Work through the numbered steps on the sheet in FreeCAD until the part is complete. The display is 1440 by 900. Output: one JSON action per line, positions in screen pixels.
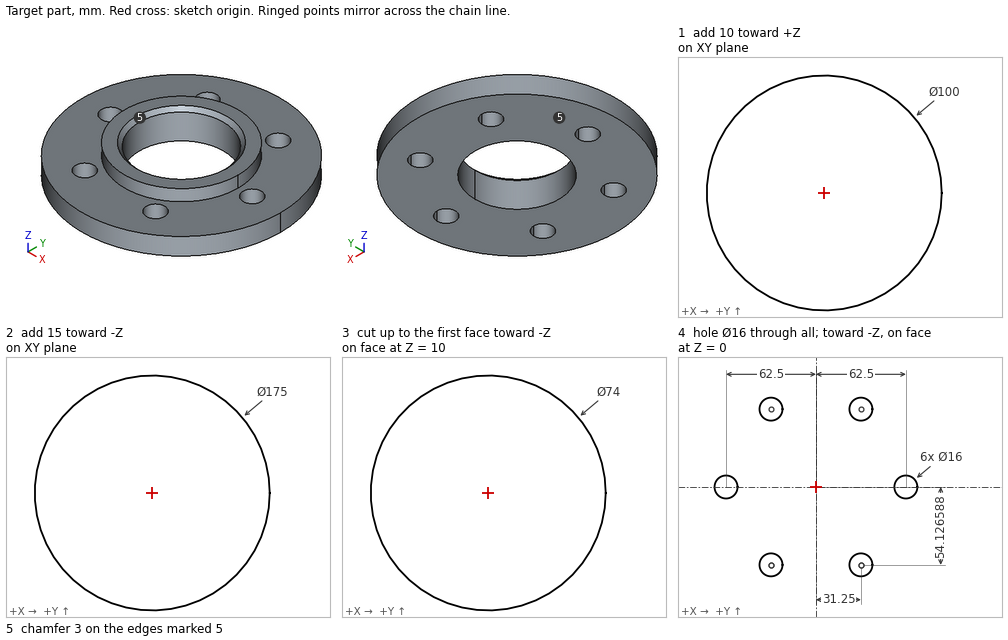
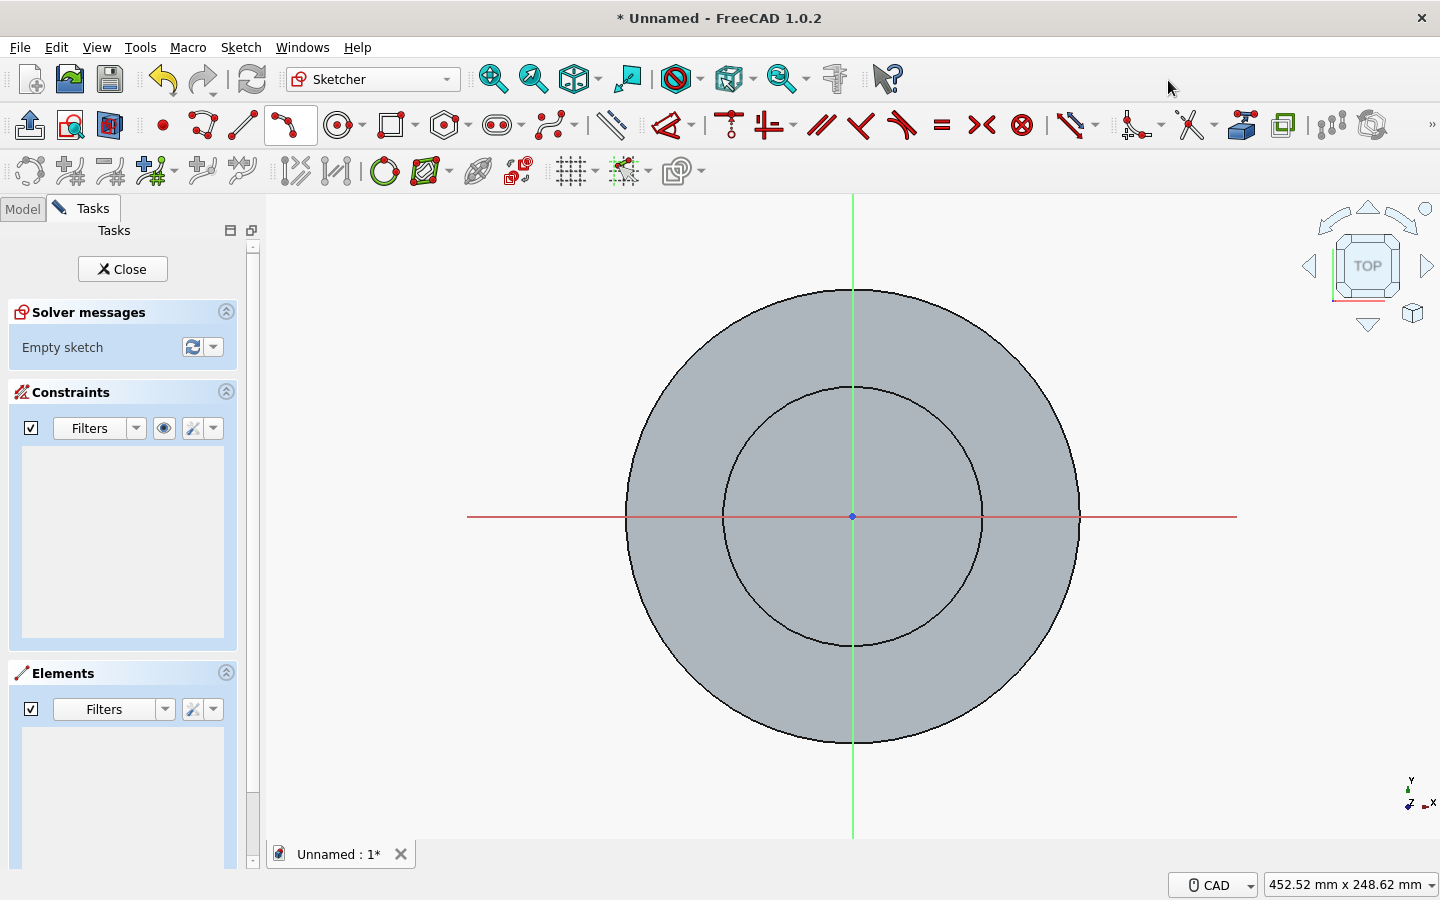
{"action": "scroll", "coordinate": [909, 517], "scroll_direction": "up", "scroll_amount": 4}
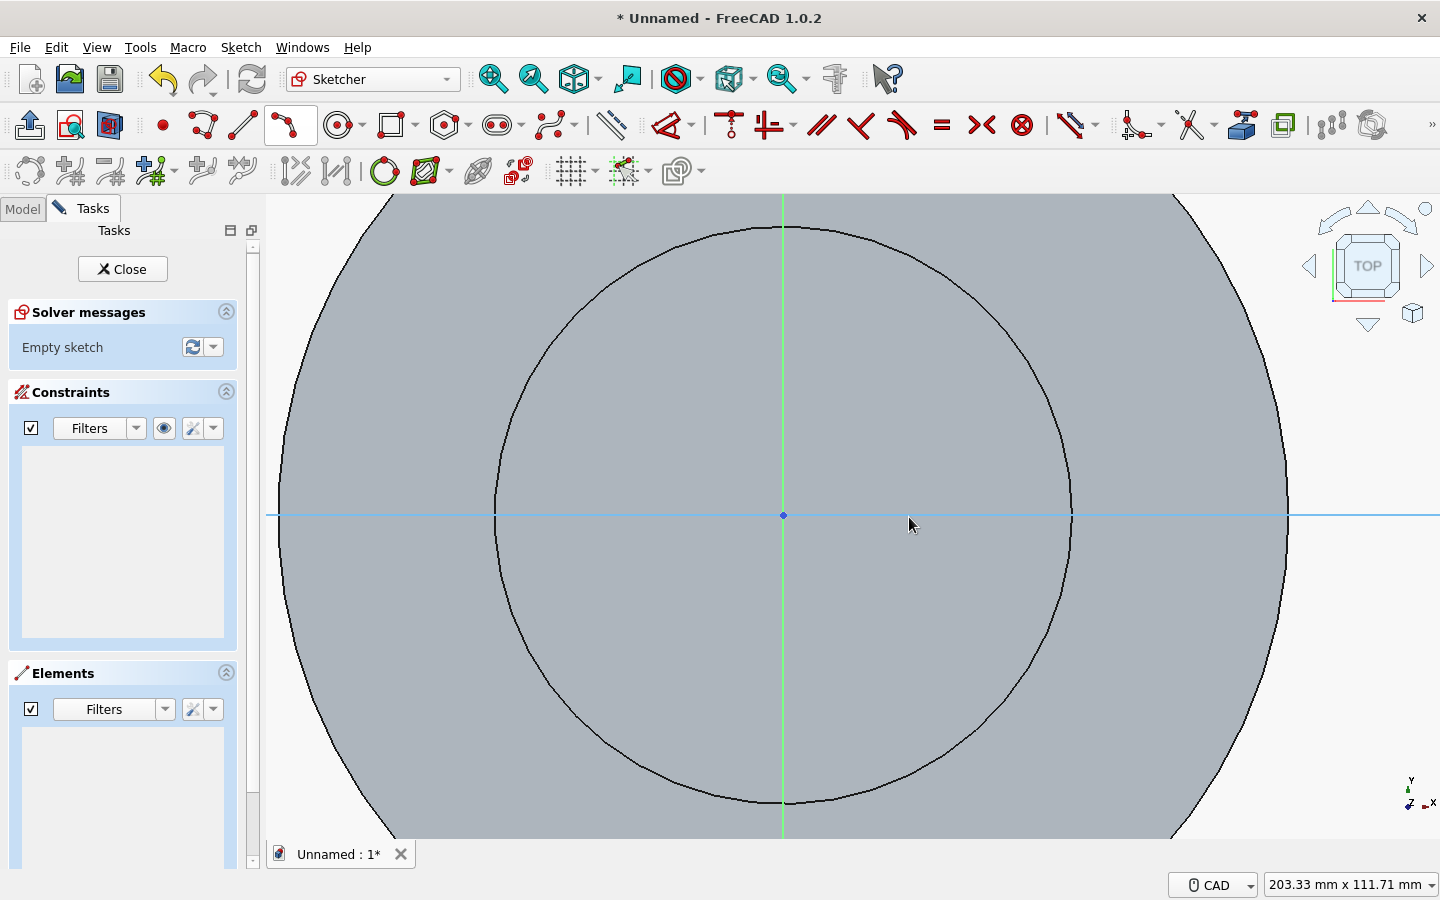
{"action": "left_click", "coordinate": [338, 126]}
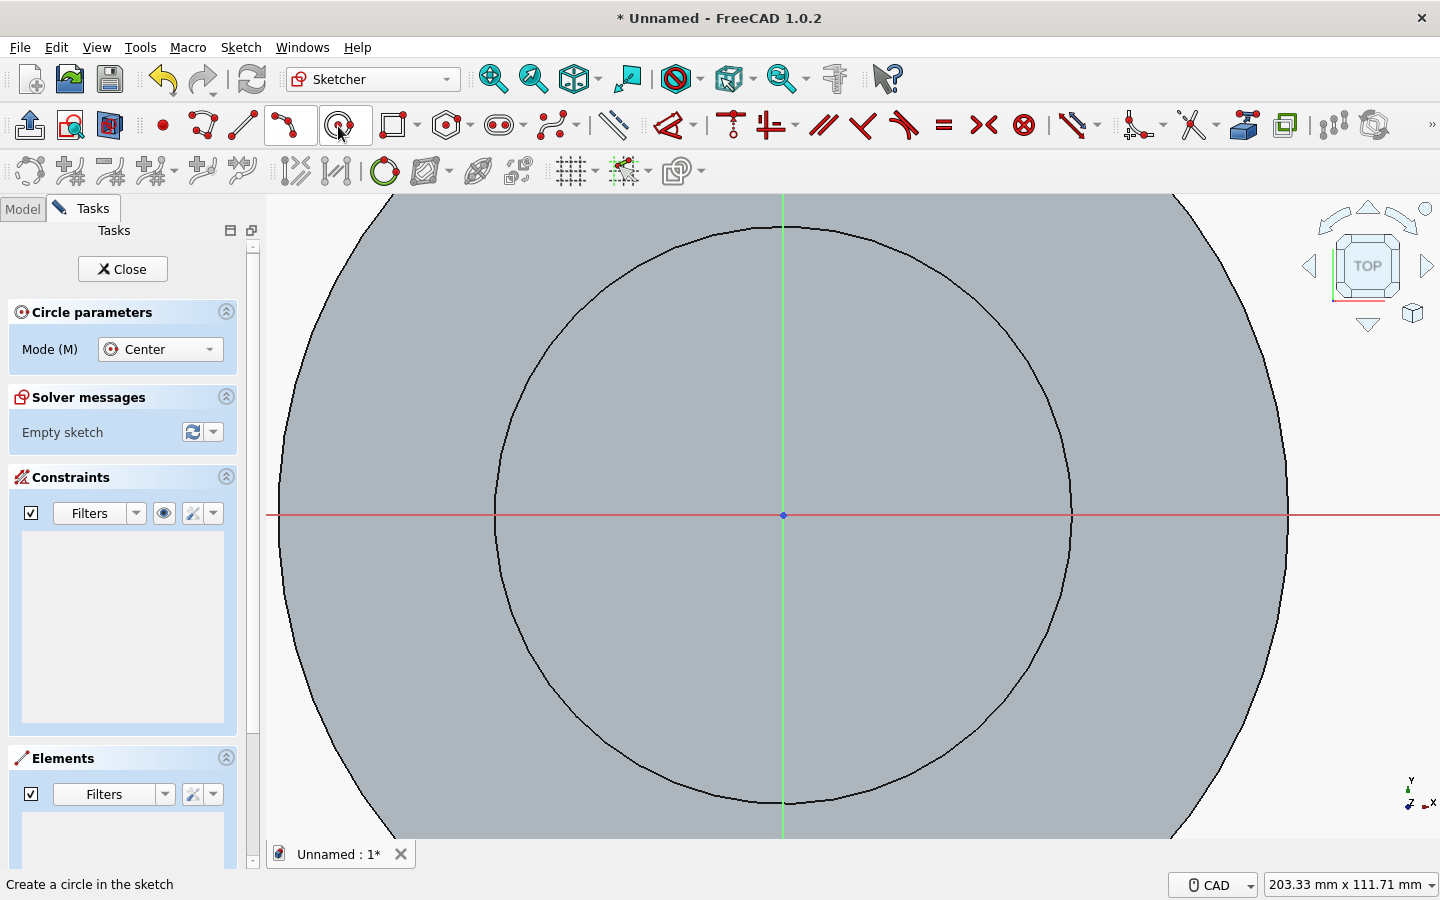
{"action": "left_click", "coordinate": [783, 515]}
{"action": "left_click", "coordinate": [934, 364]}
{"action": "key", "text": "Escape"}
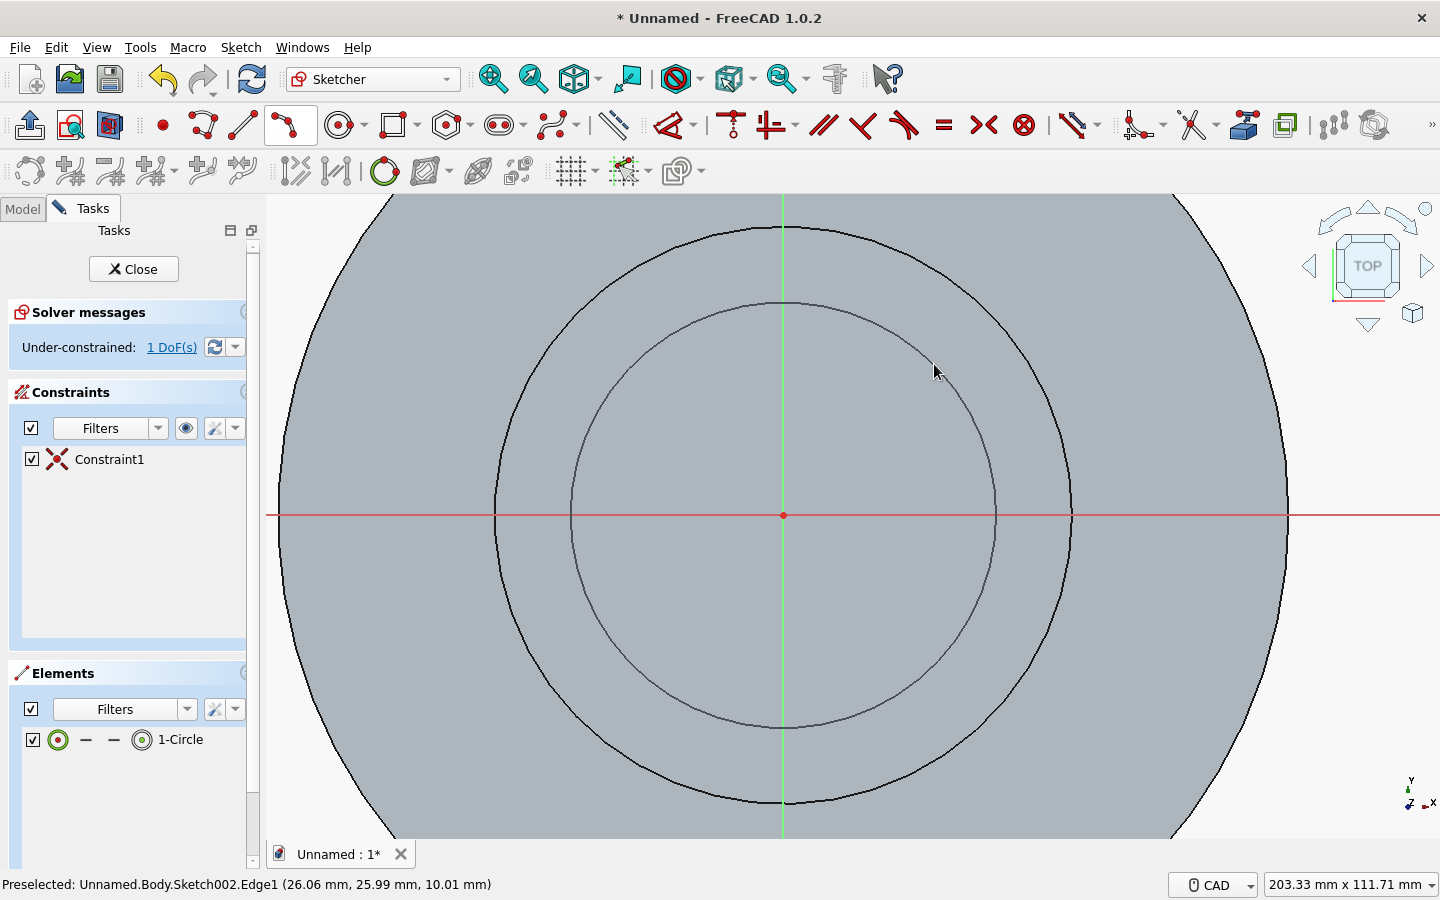
{"action": "left_click", "coordinate": [668, 126]}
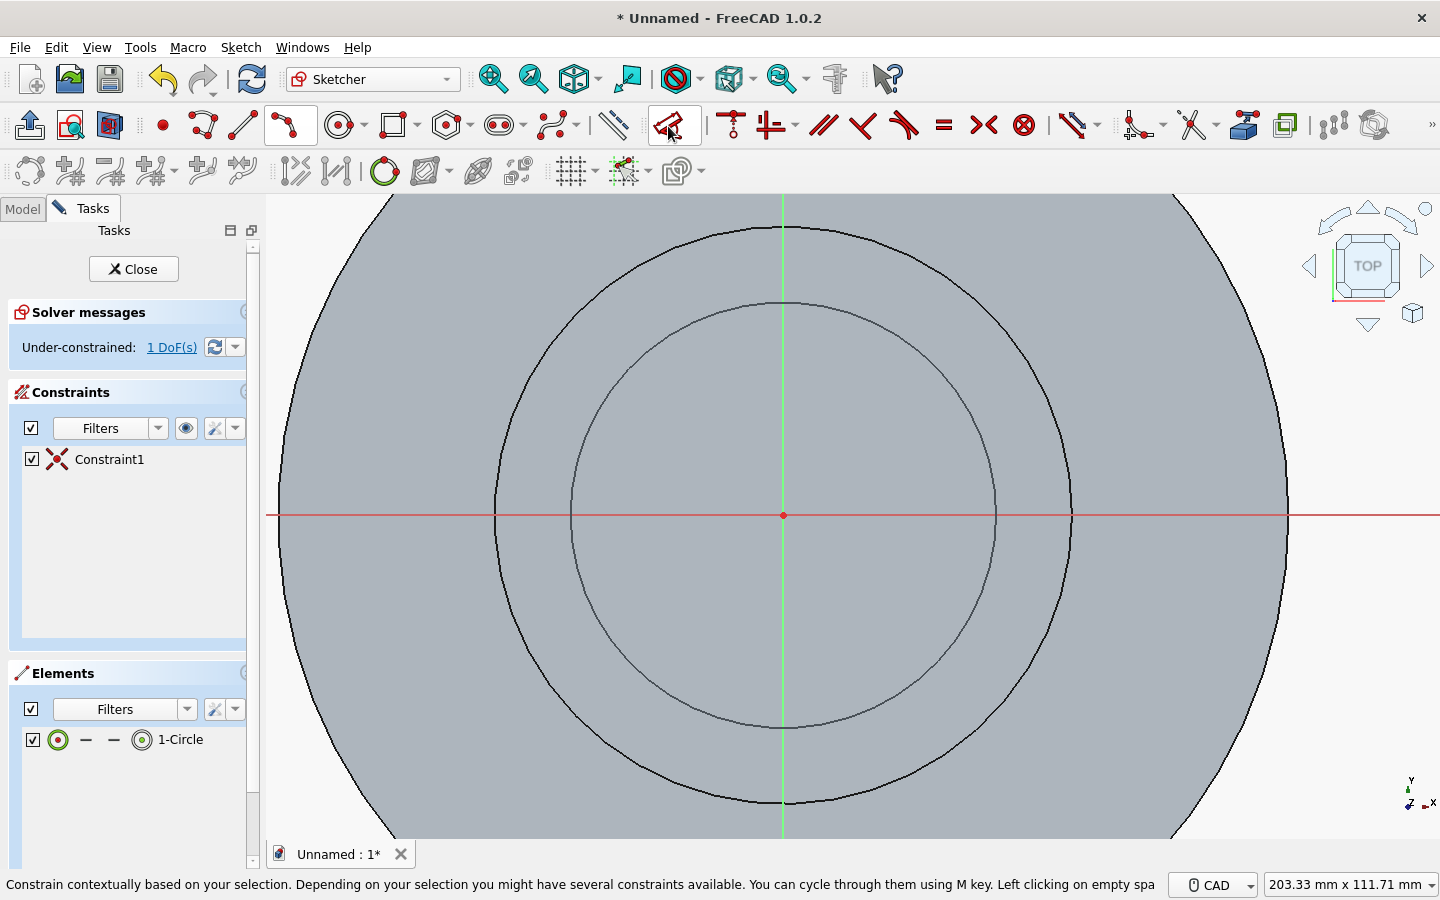
{"action": "left_click", "coordinate": [933, 364]}
{"action": "left_click", "coordinate": [956, 341]}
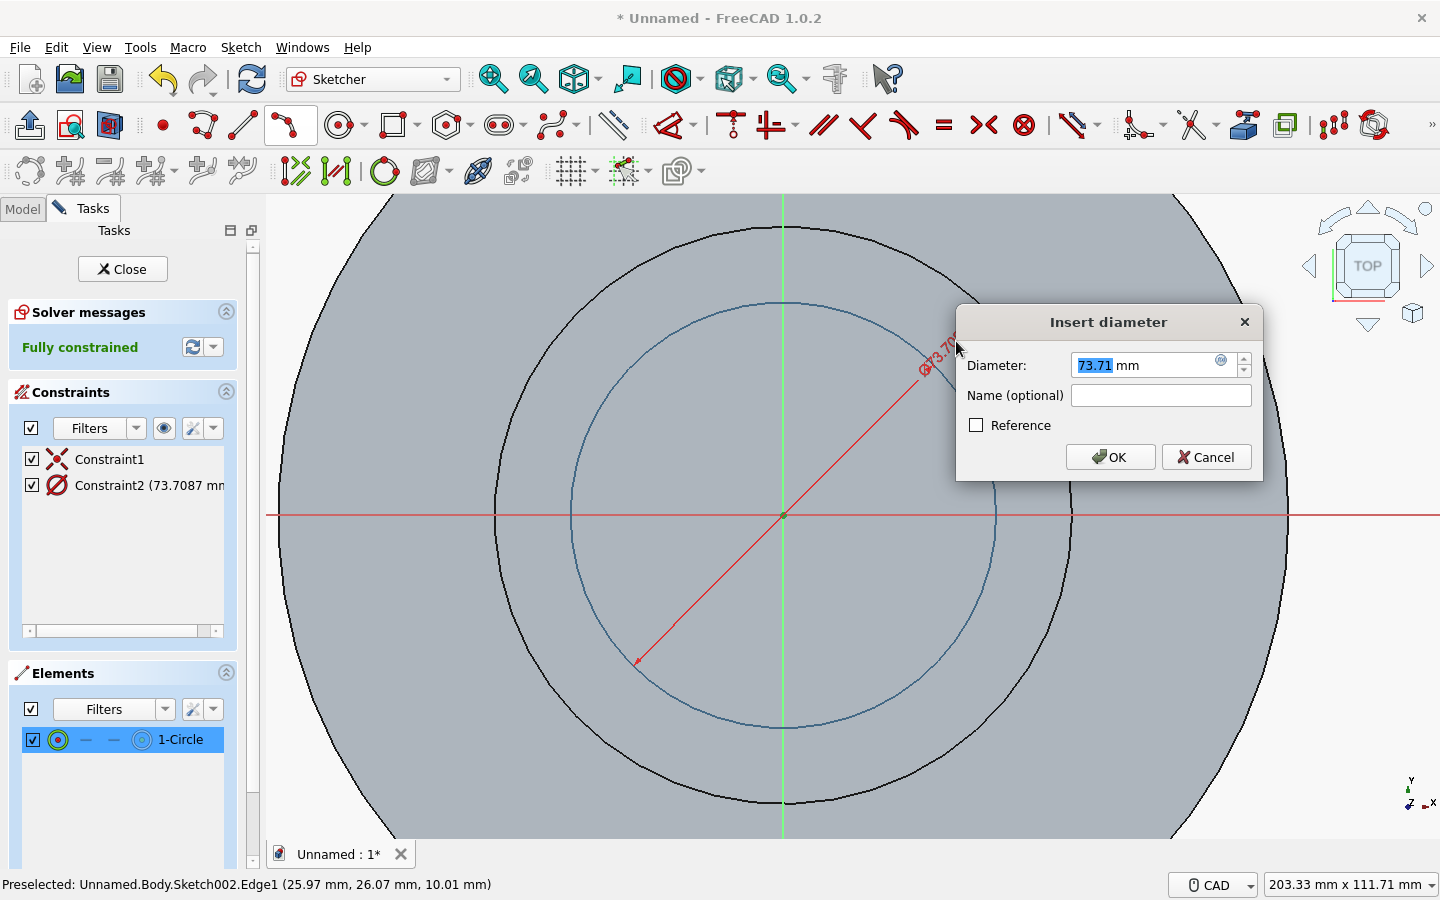
{"action": "type", "text": "74"}
{"action": "key", "text": "Return"}
{"action": "key", "text": "Escape"}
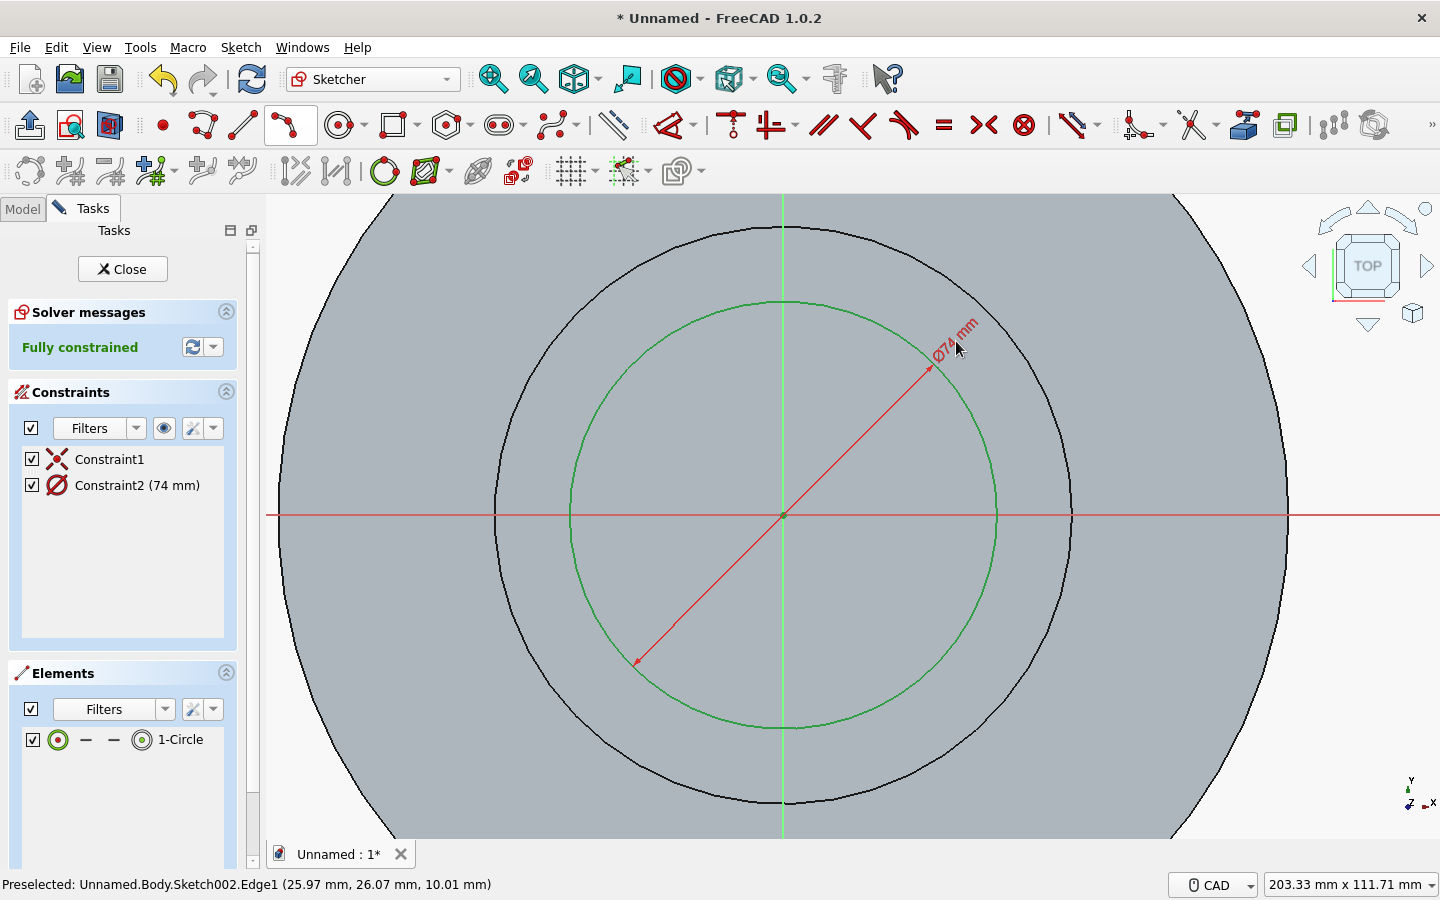
{"action": "left_click", "coordinate": [123, 269]}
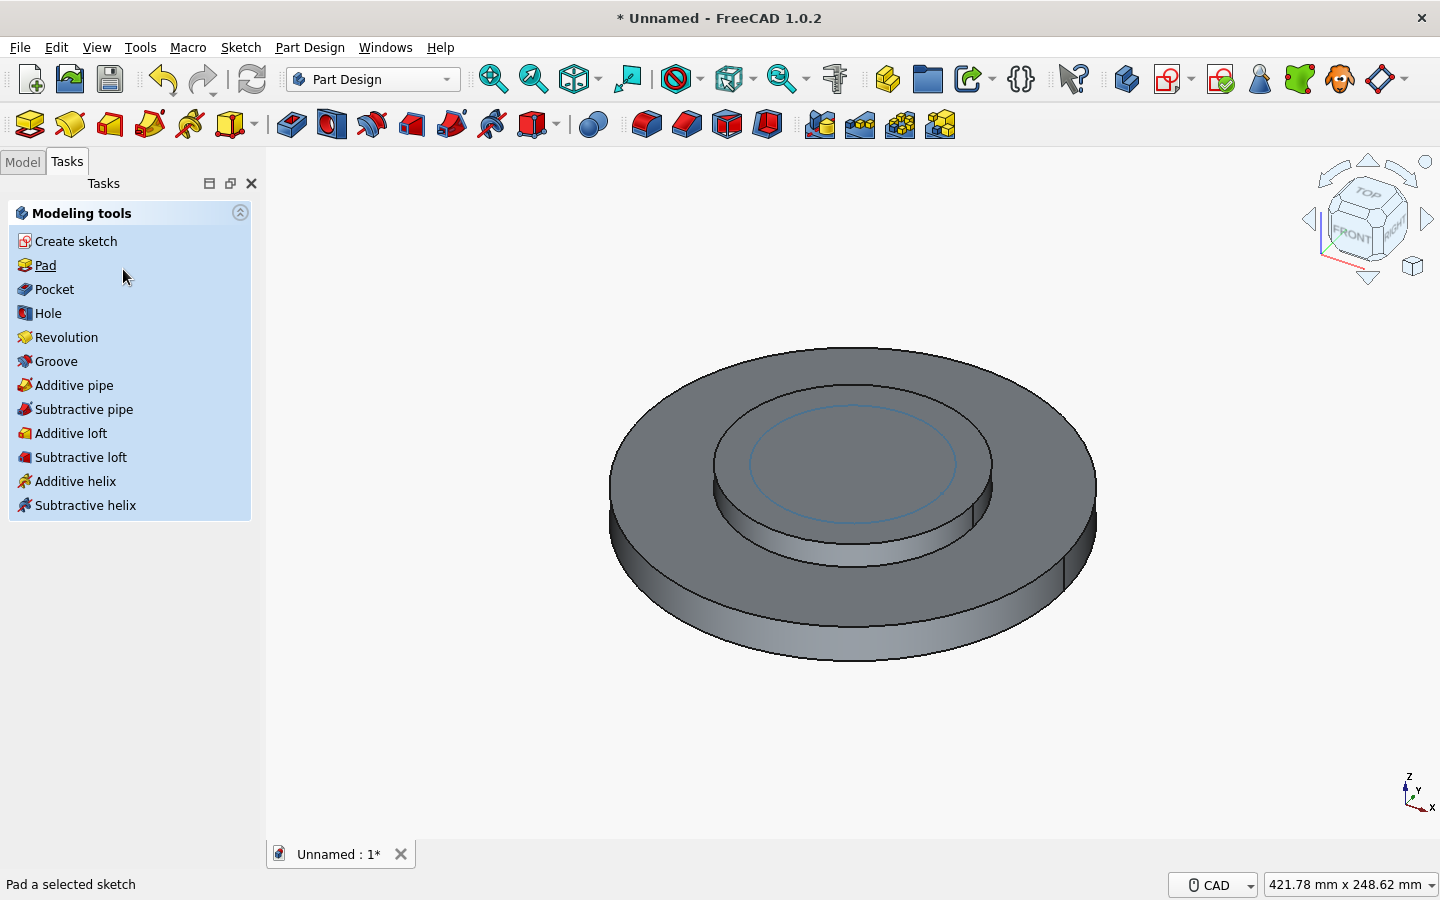
{"action": "left_click", "coordinate": [292, 124]}